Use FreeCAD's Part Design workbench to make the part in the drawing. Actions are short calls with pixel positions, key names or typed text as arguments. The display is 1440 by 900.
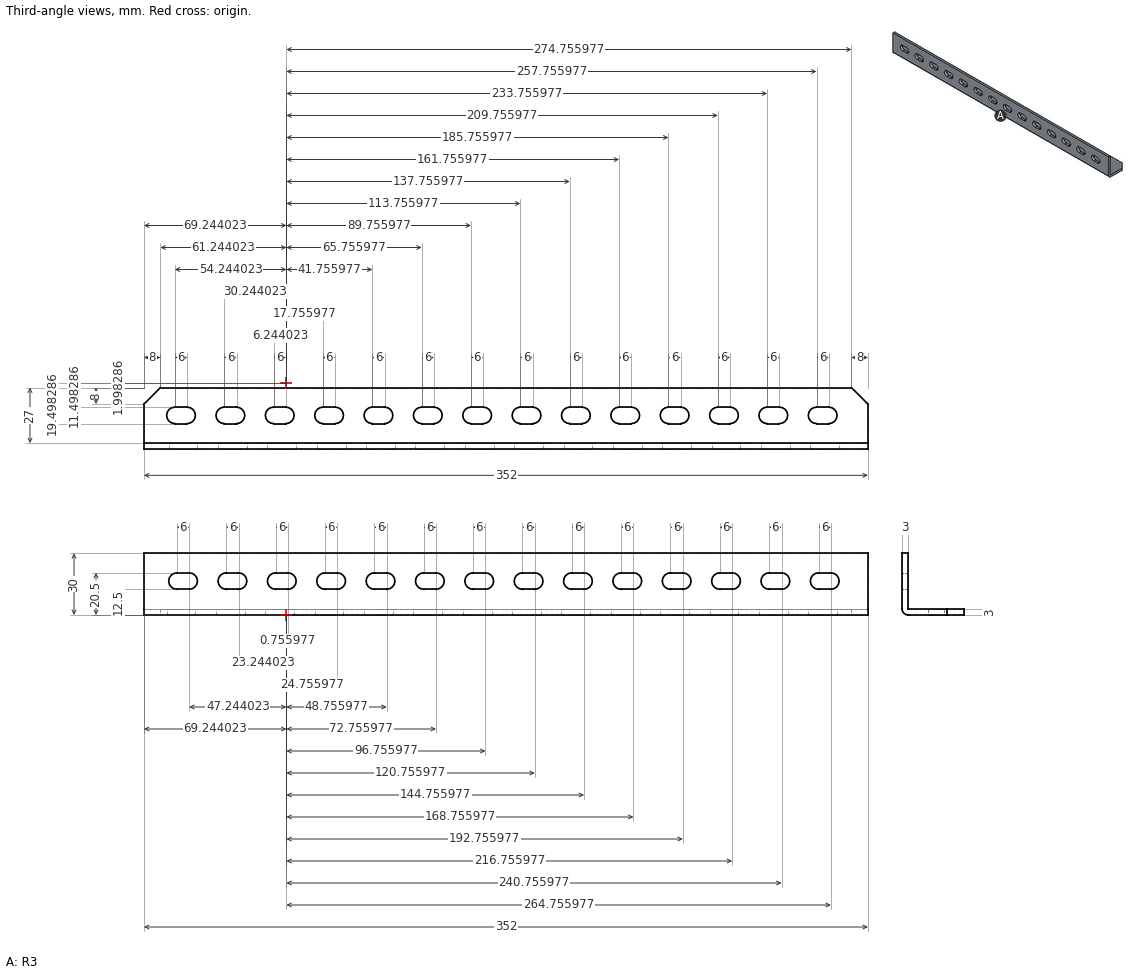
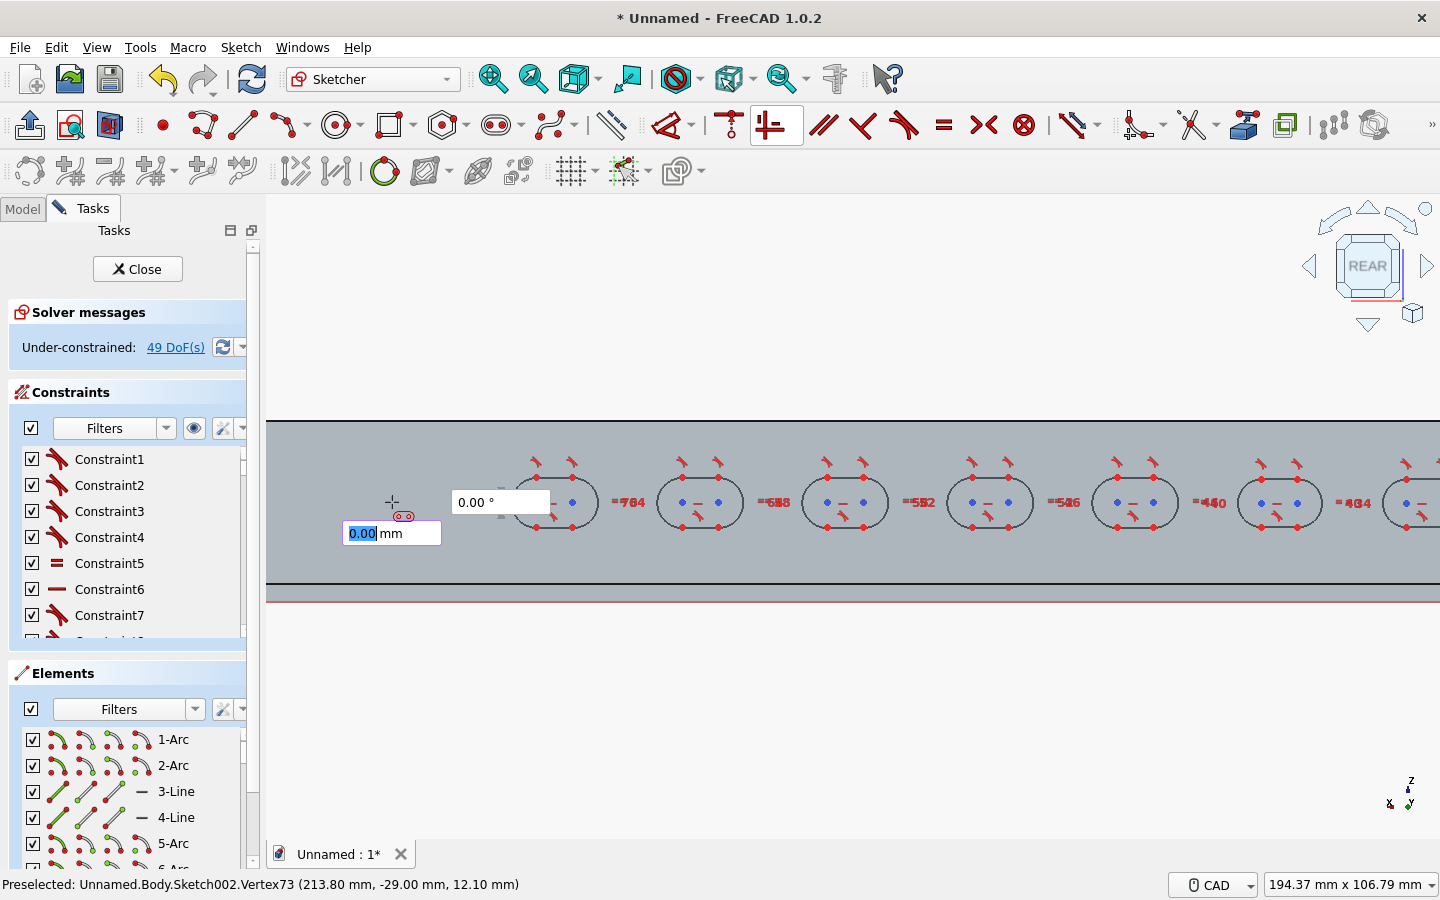
click(428, 502)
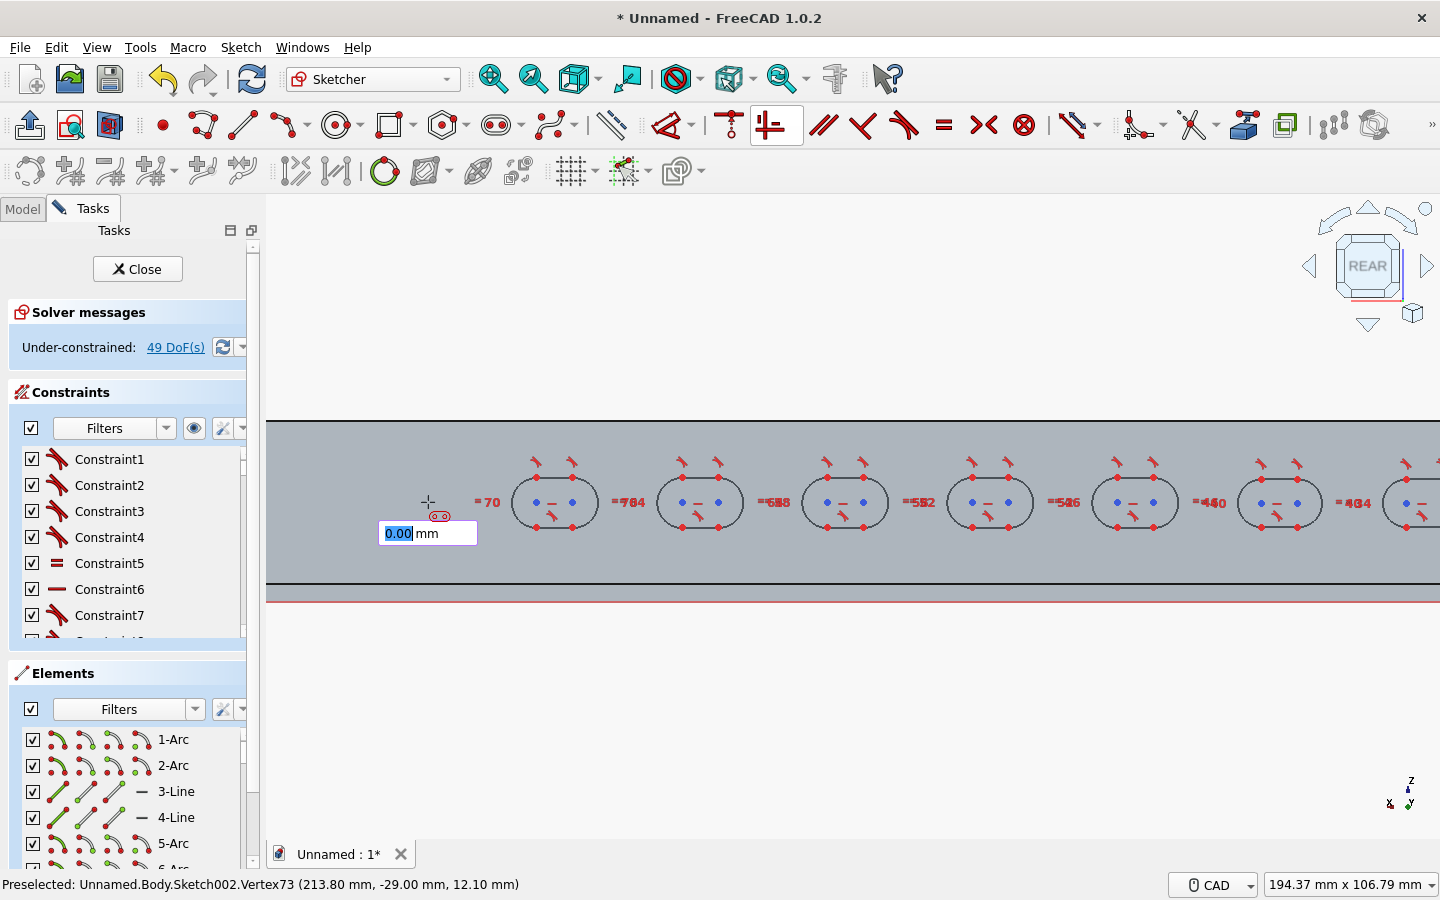
click(410, 527)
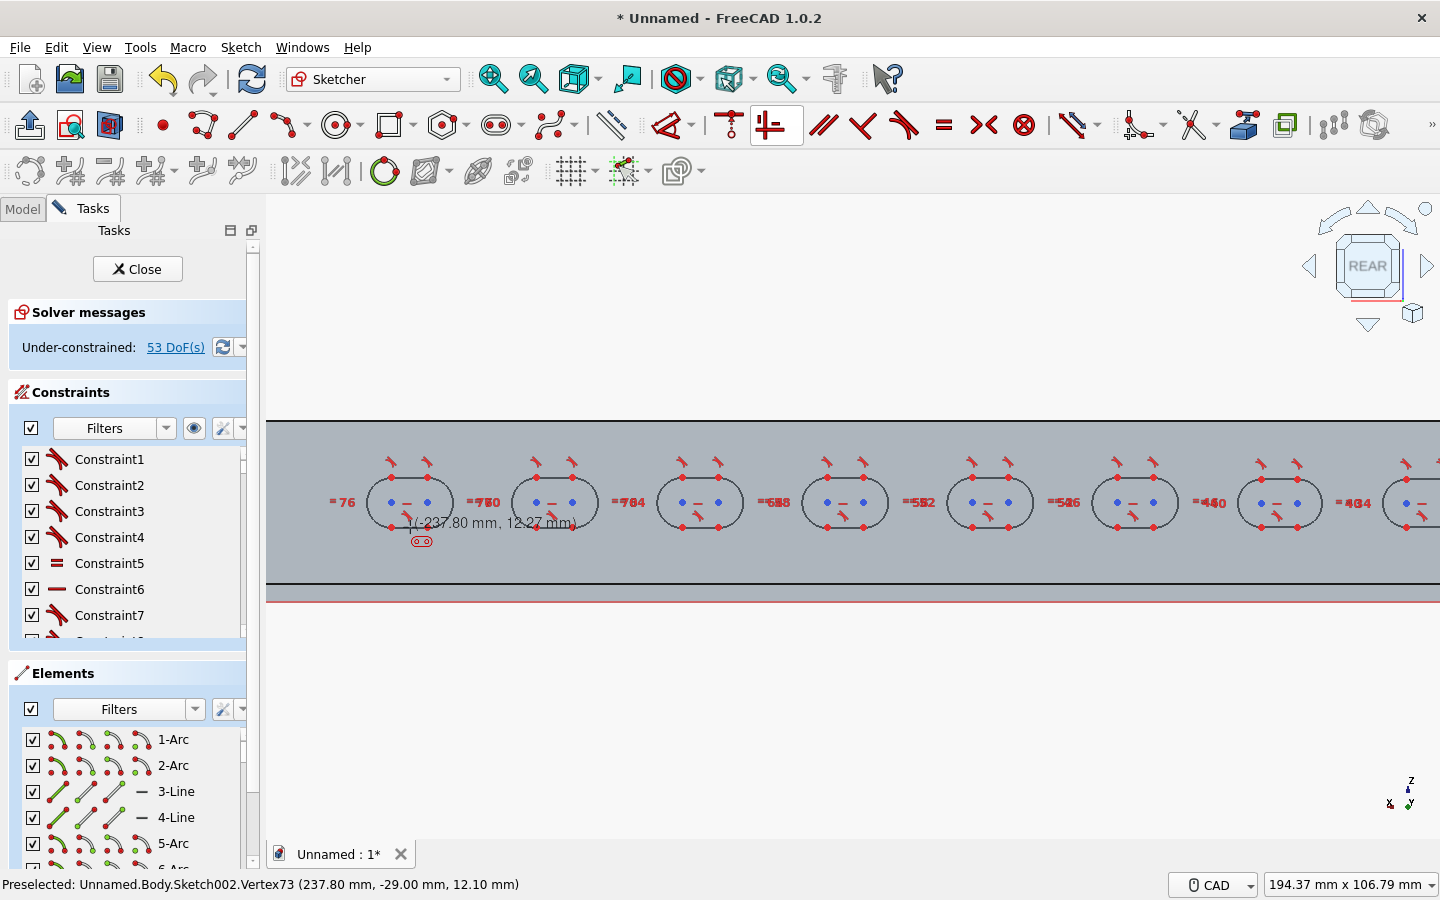
scroll(538, 503, down, 5)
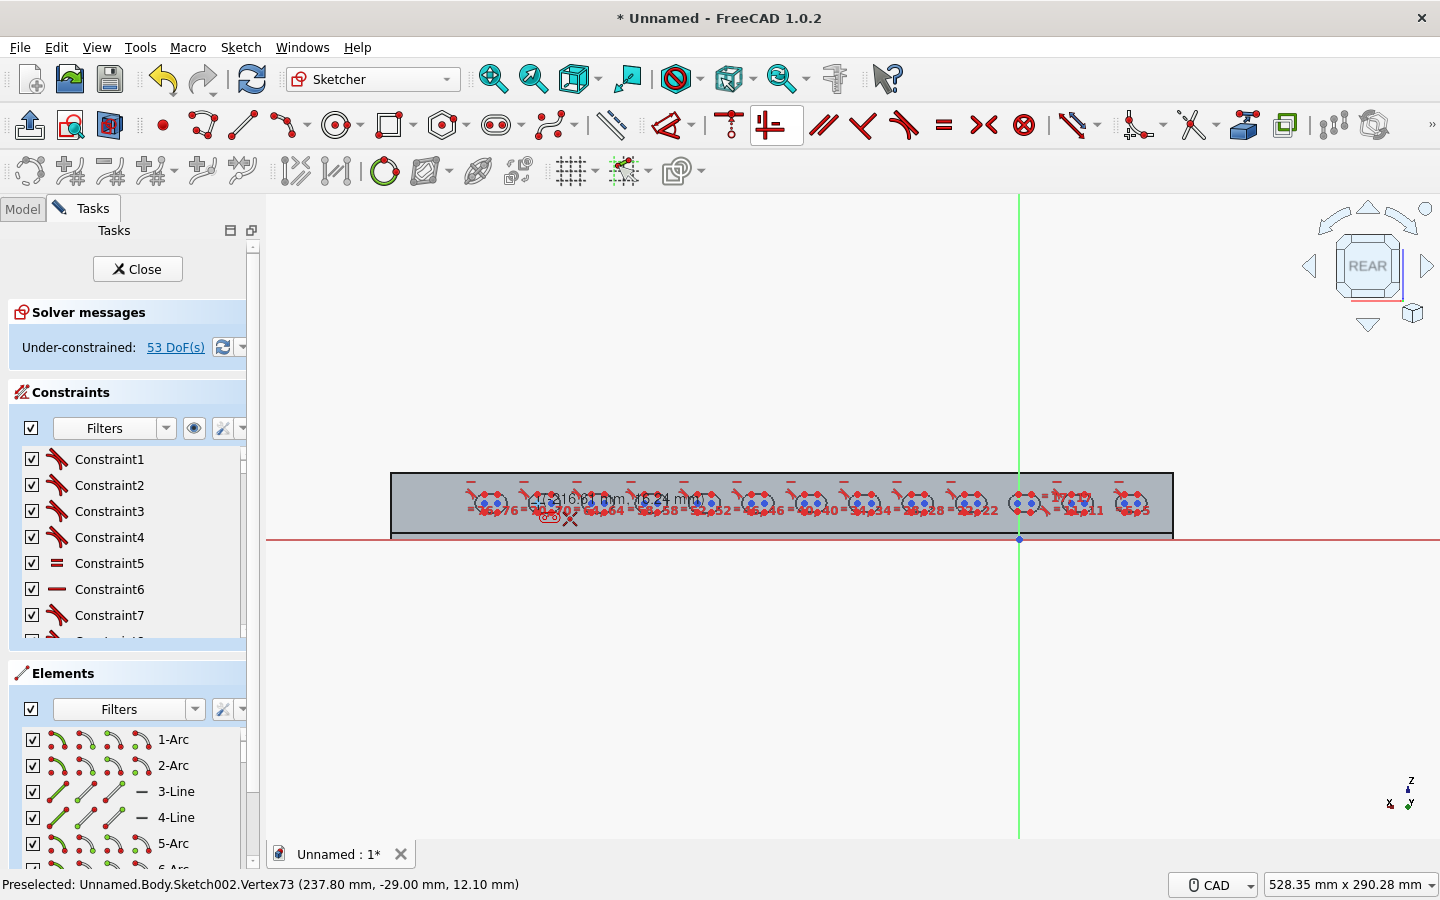
scroll(431, 503, up, 5)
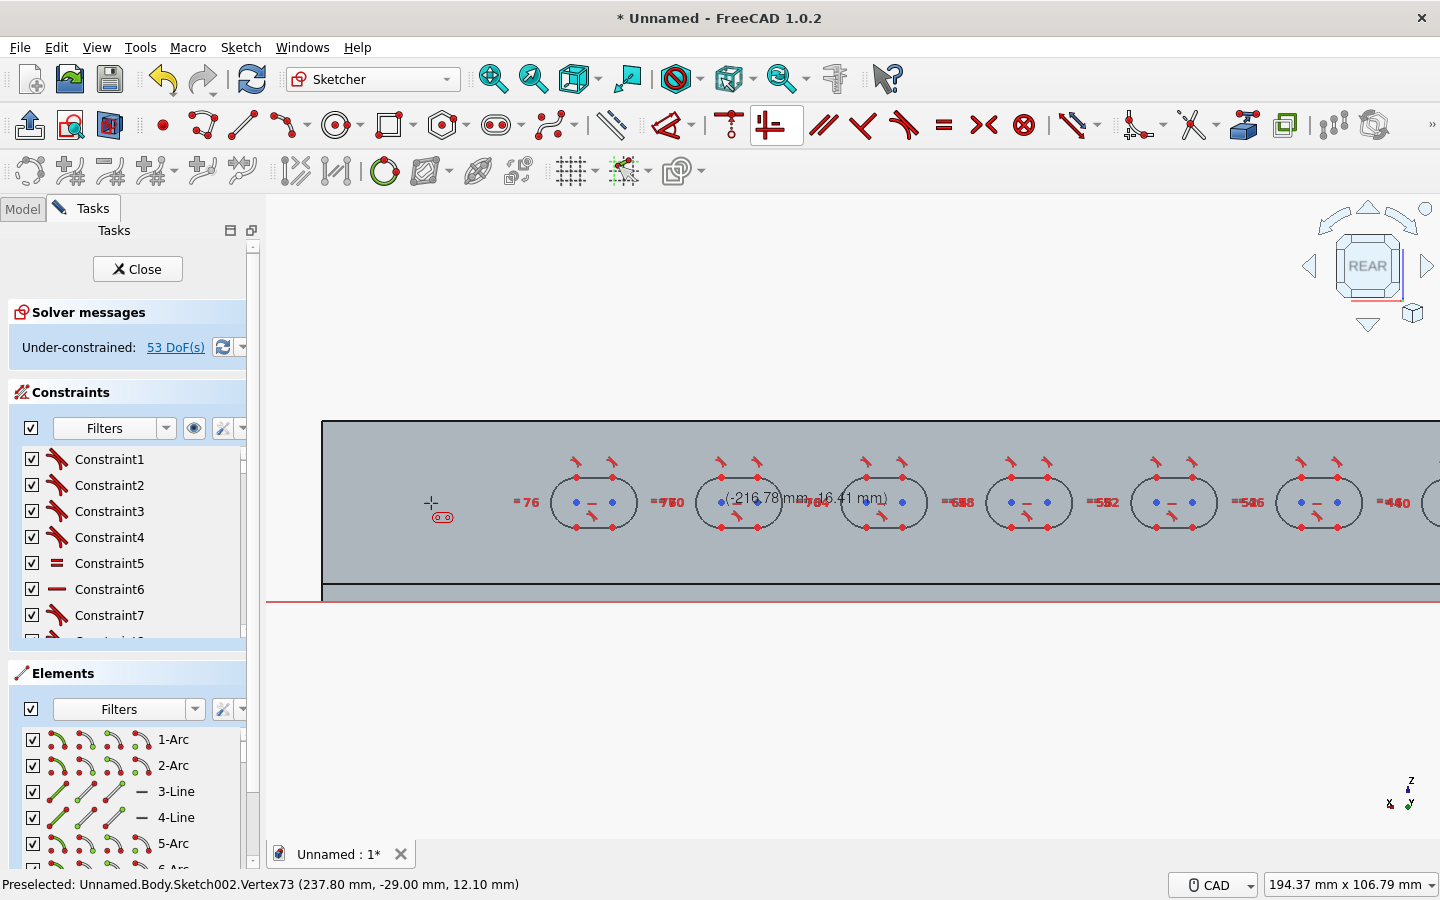
click(431, 502)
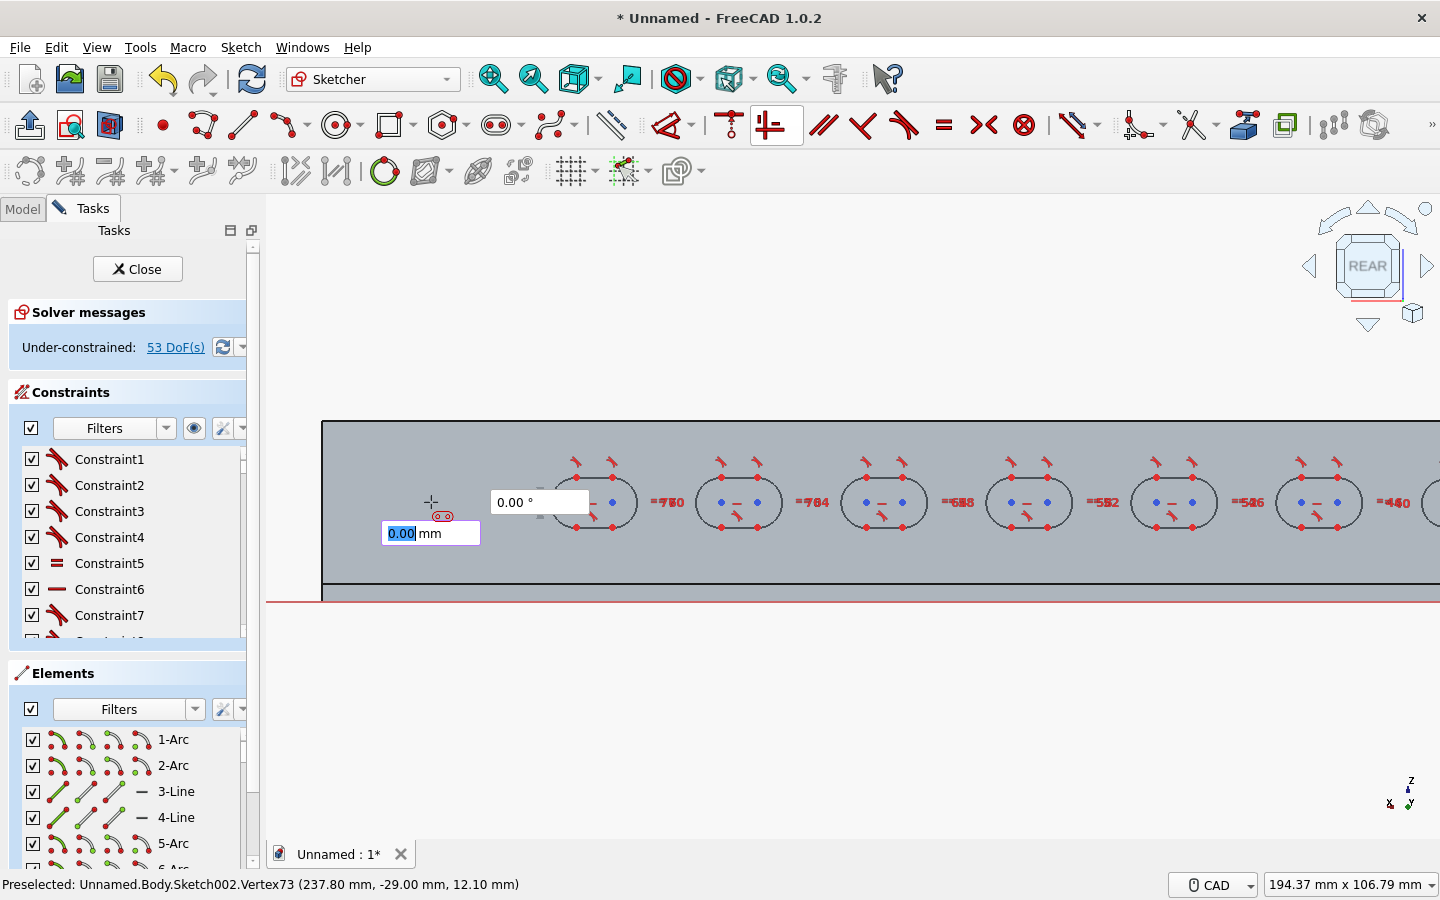
click(467, 502)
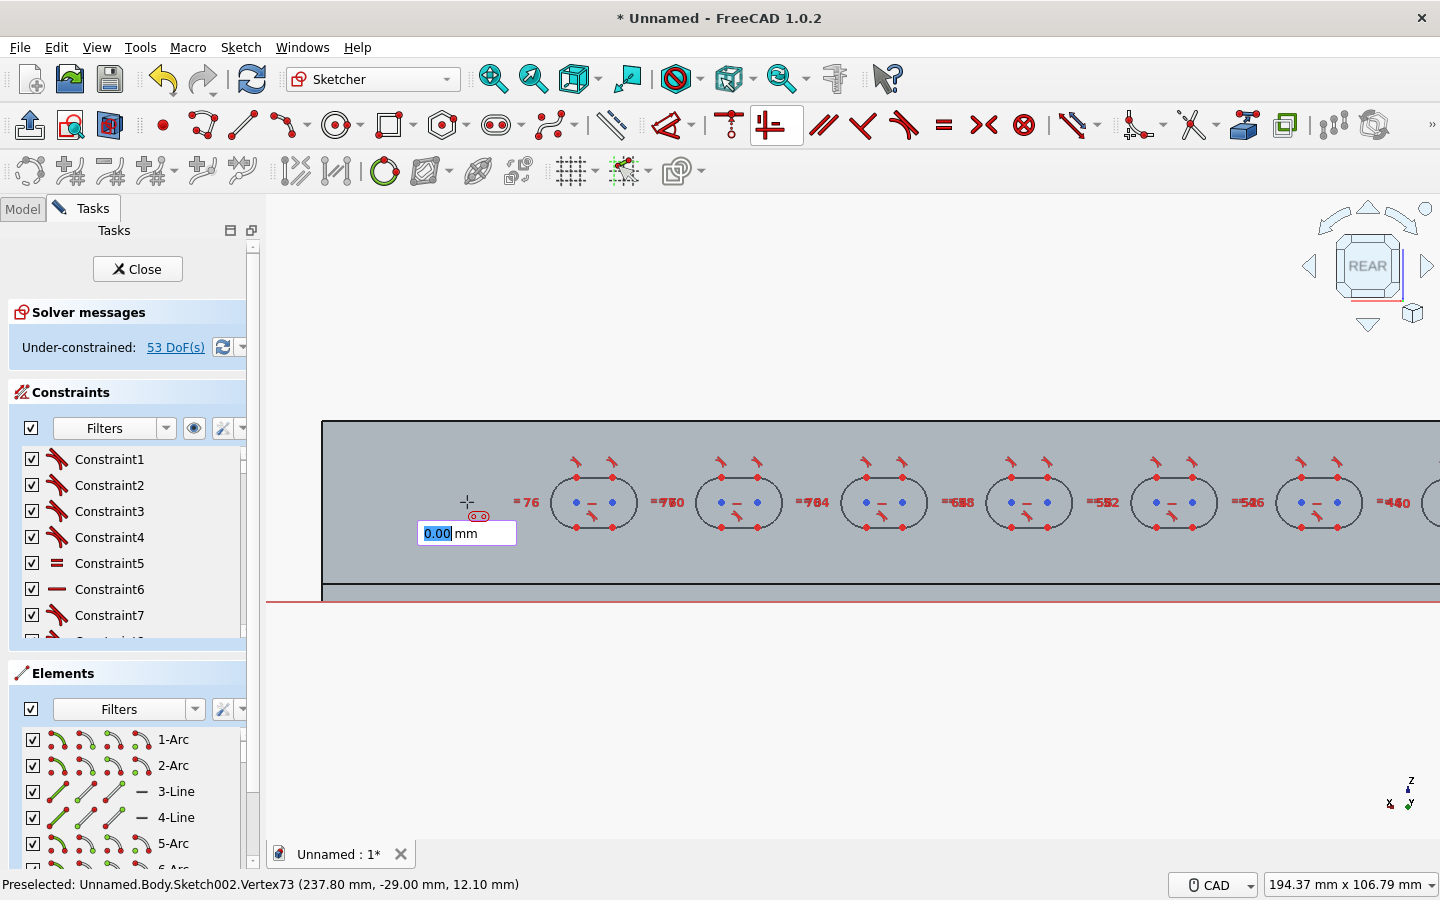
click(449, 527)
key(Escape)